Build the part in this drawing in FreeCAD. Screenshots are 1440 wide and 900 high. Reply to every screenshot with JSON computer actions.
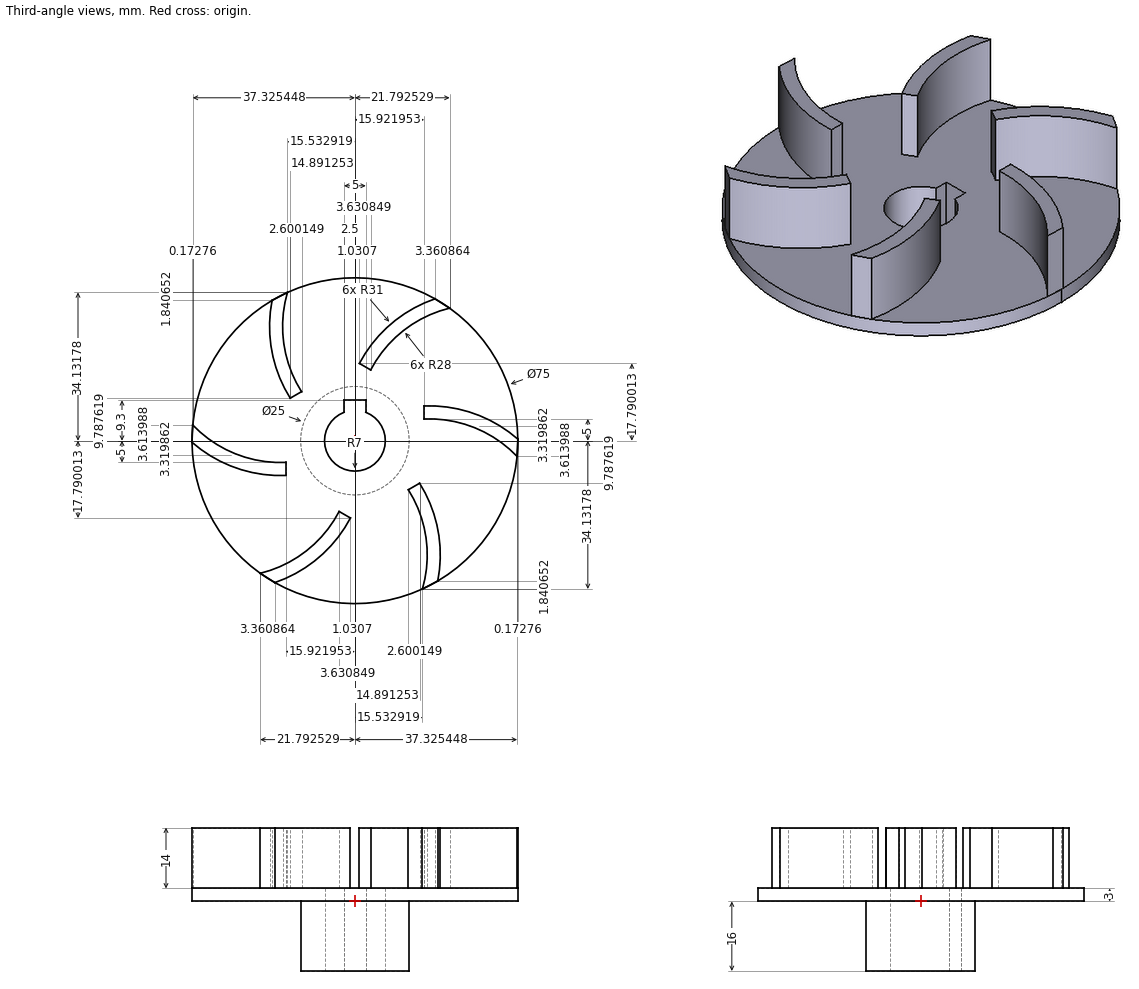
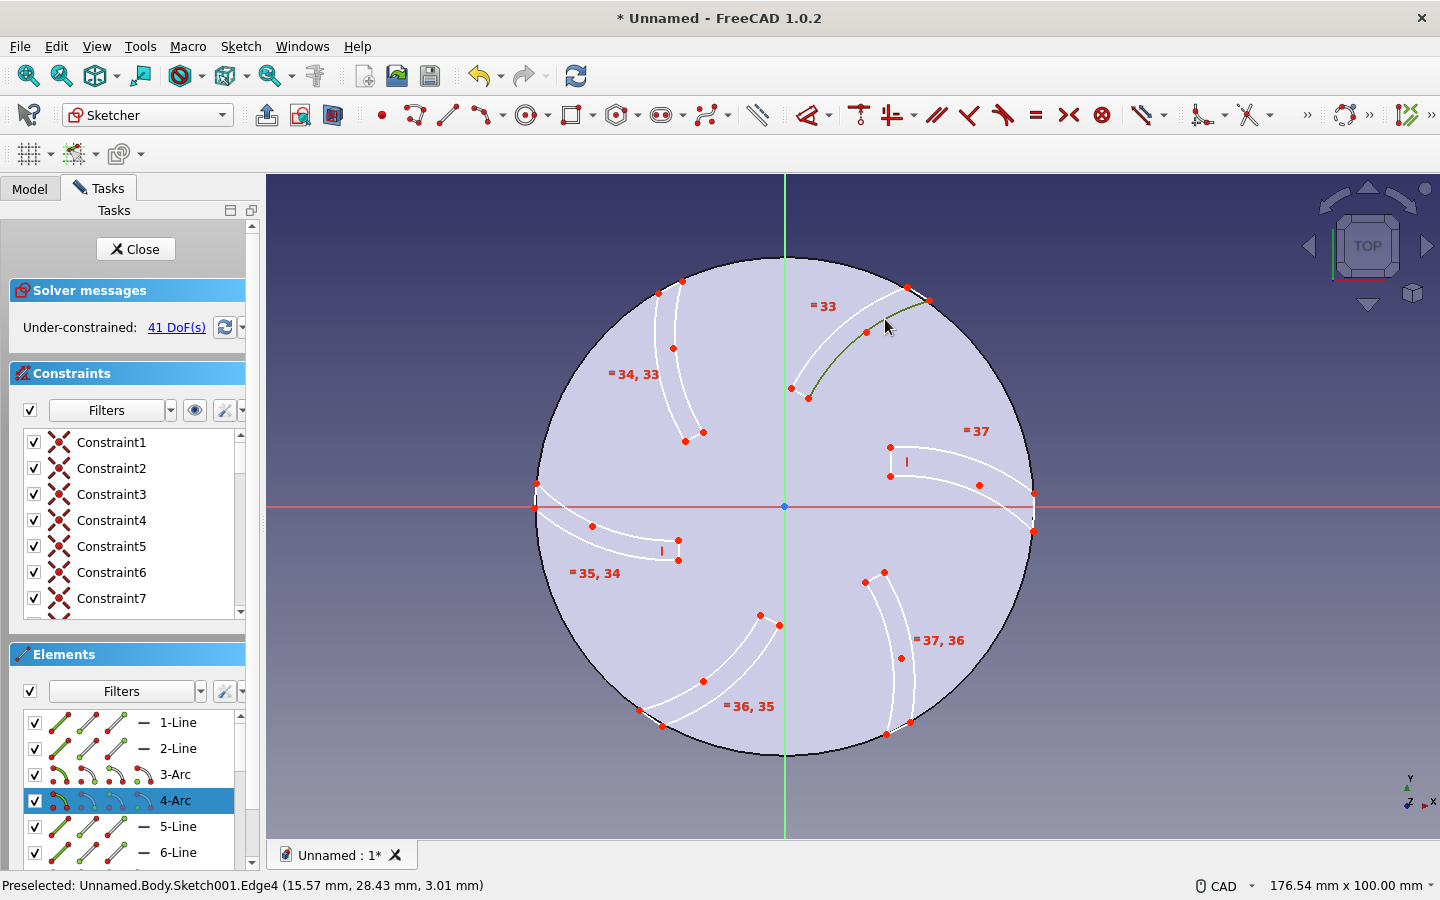
{"action": "left_click", "coordinate": [675, 327]}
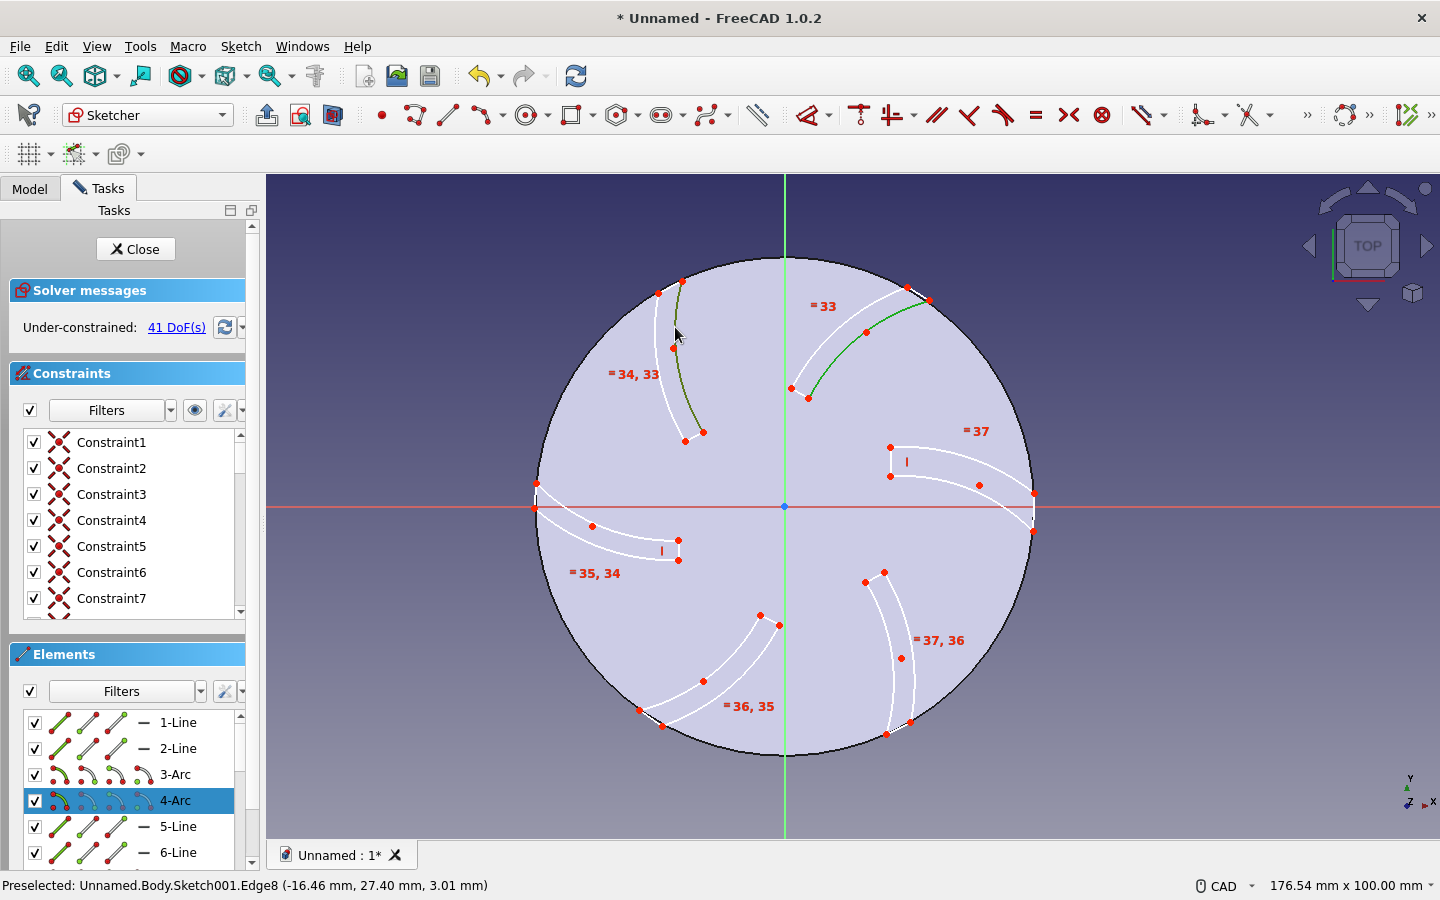
{"action": "left_click", "coordinate": [632, 536]}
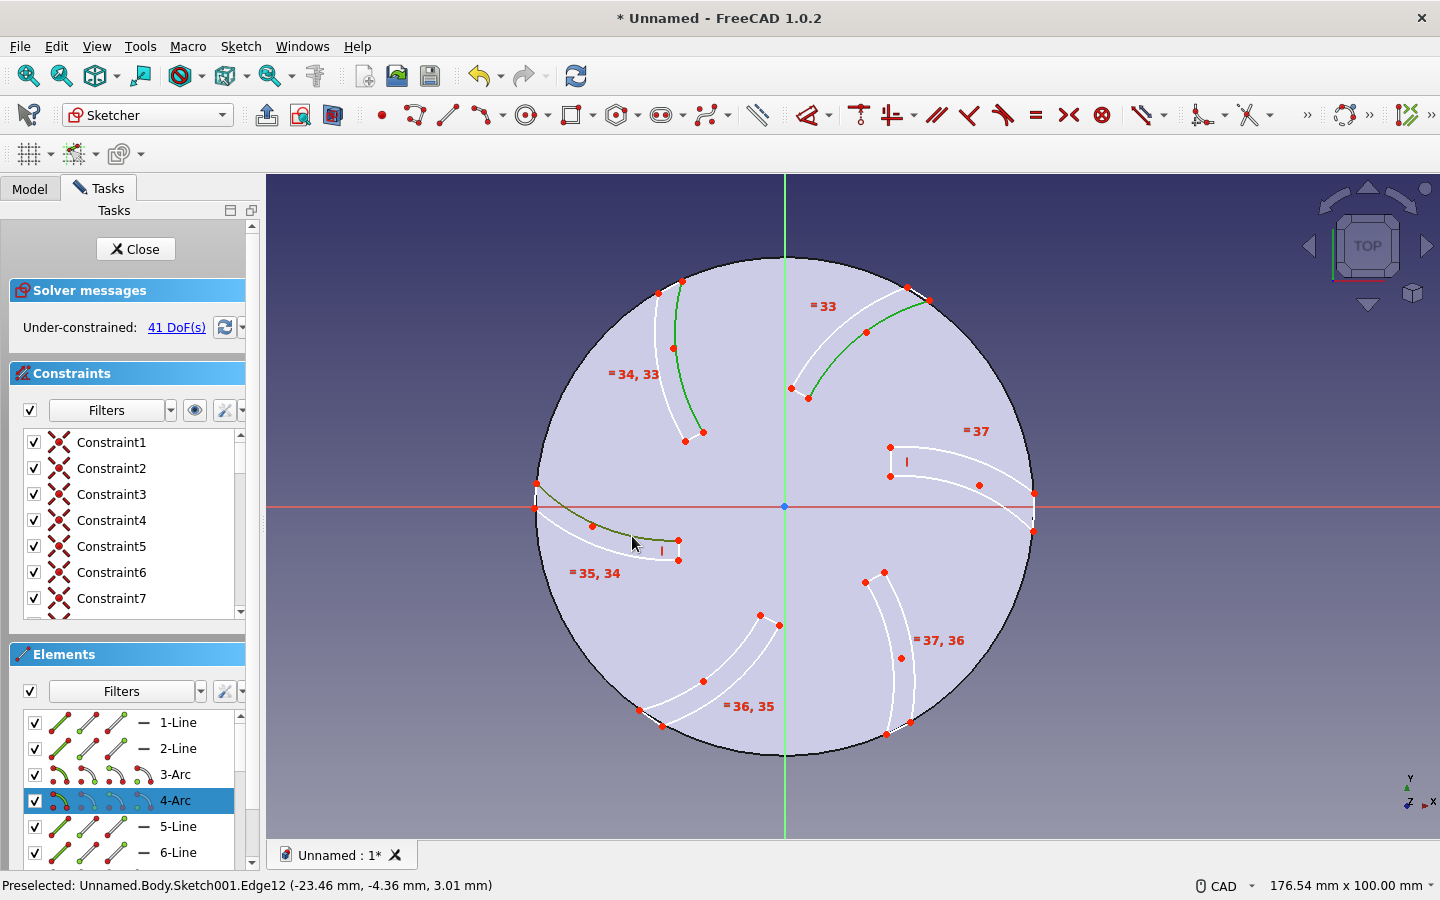
{"action": "left_click", "coordinate": [684, 693]}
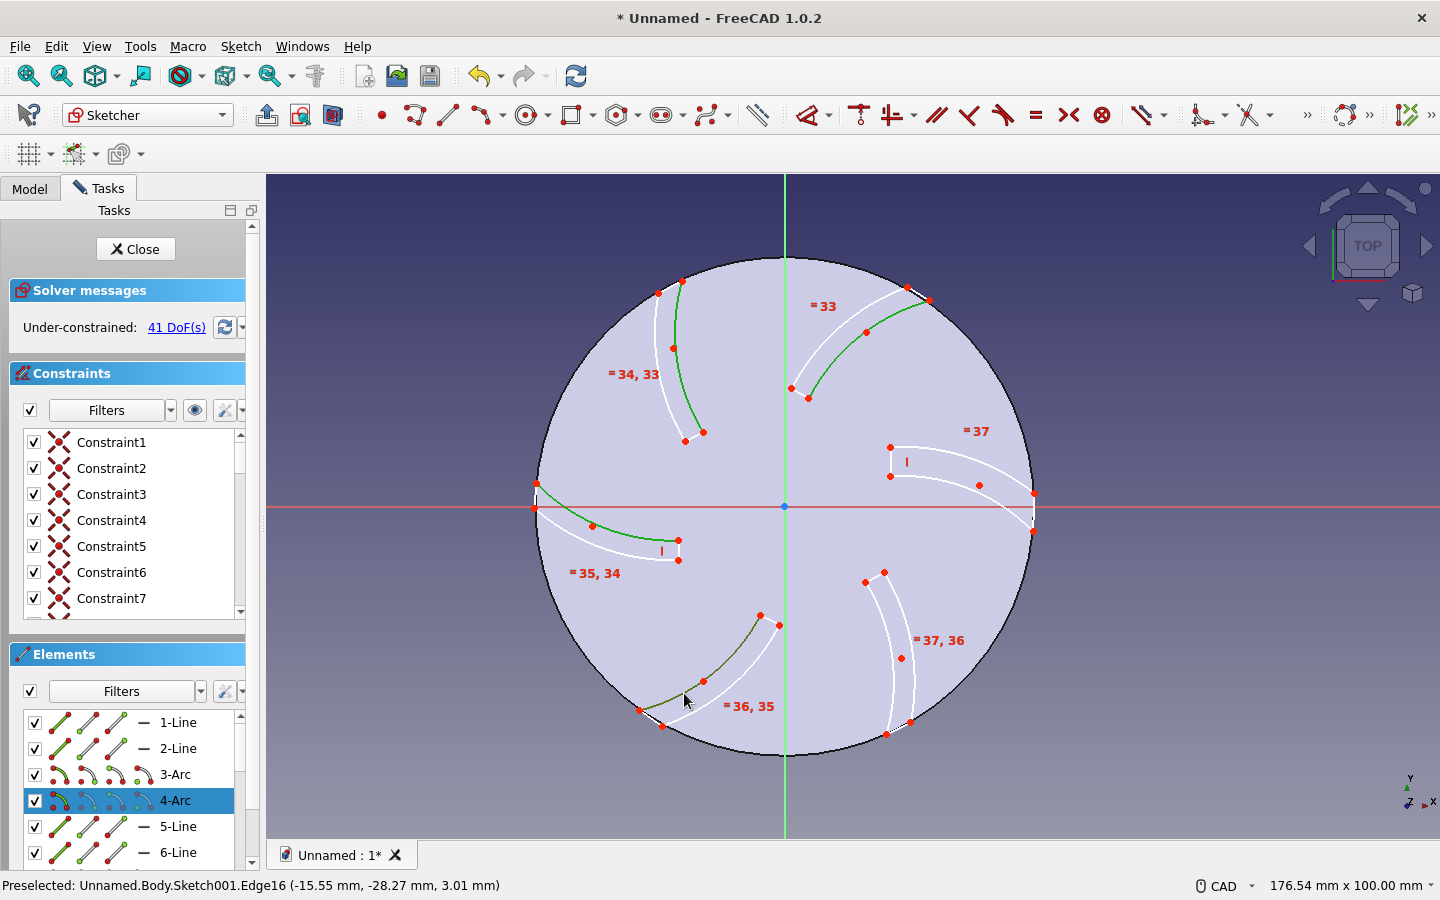
{"action": "left_click", "coordinate": [894, 688]}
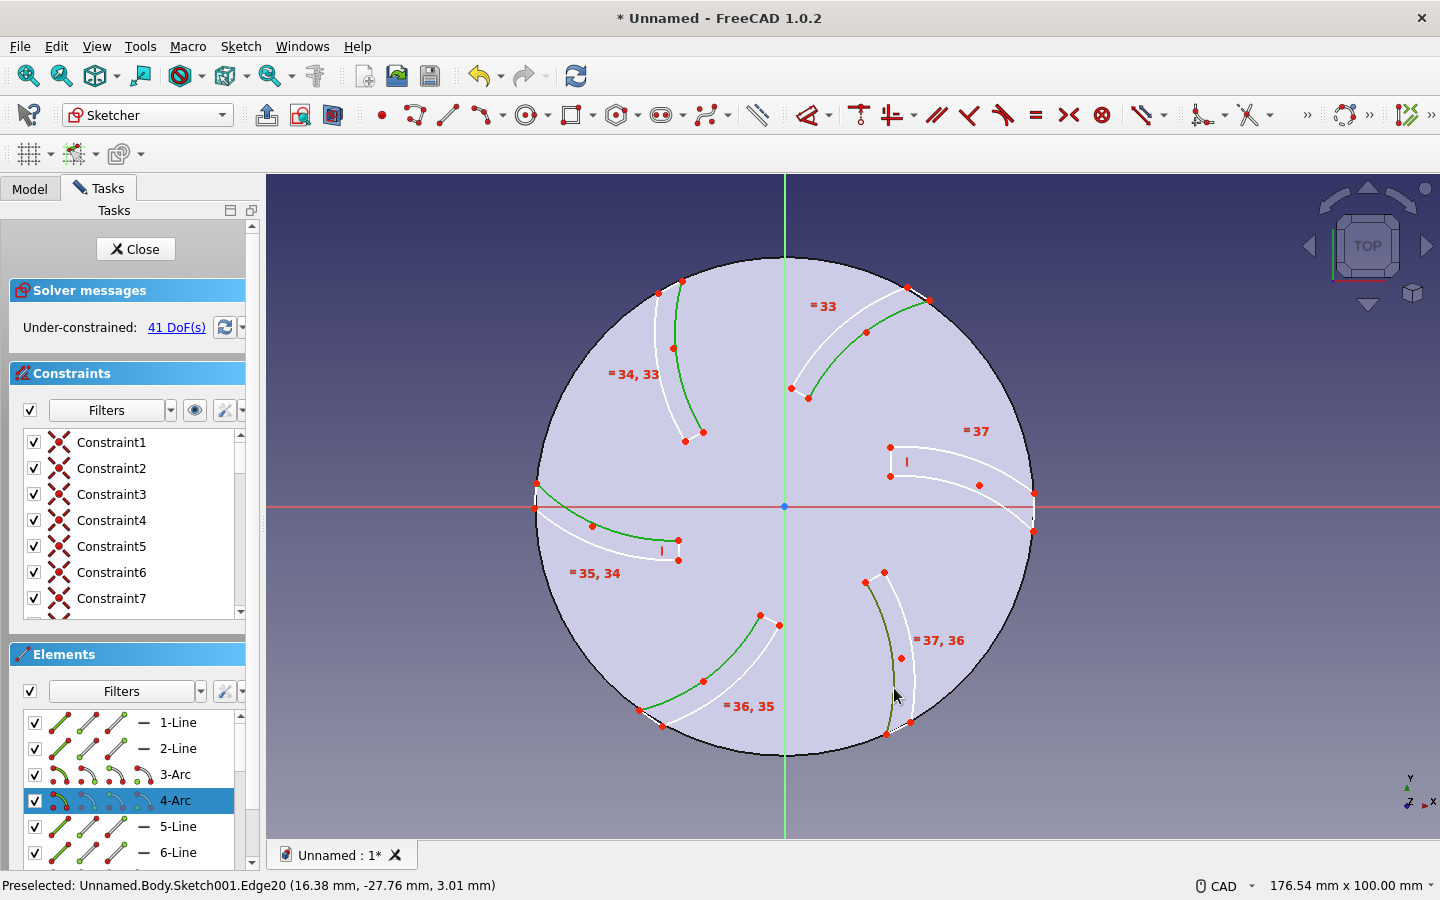
{"action": "left_click", "coordinate": [938, 480]}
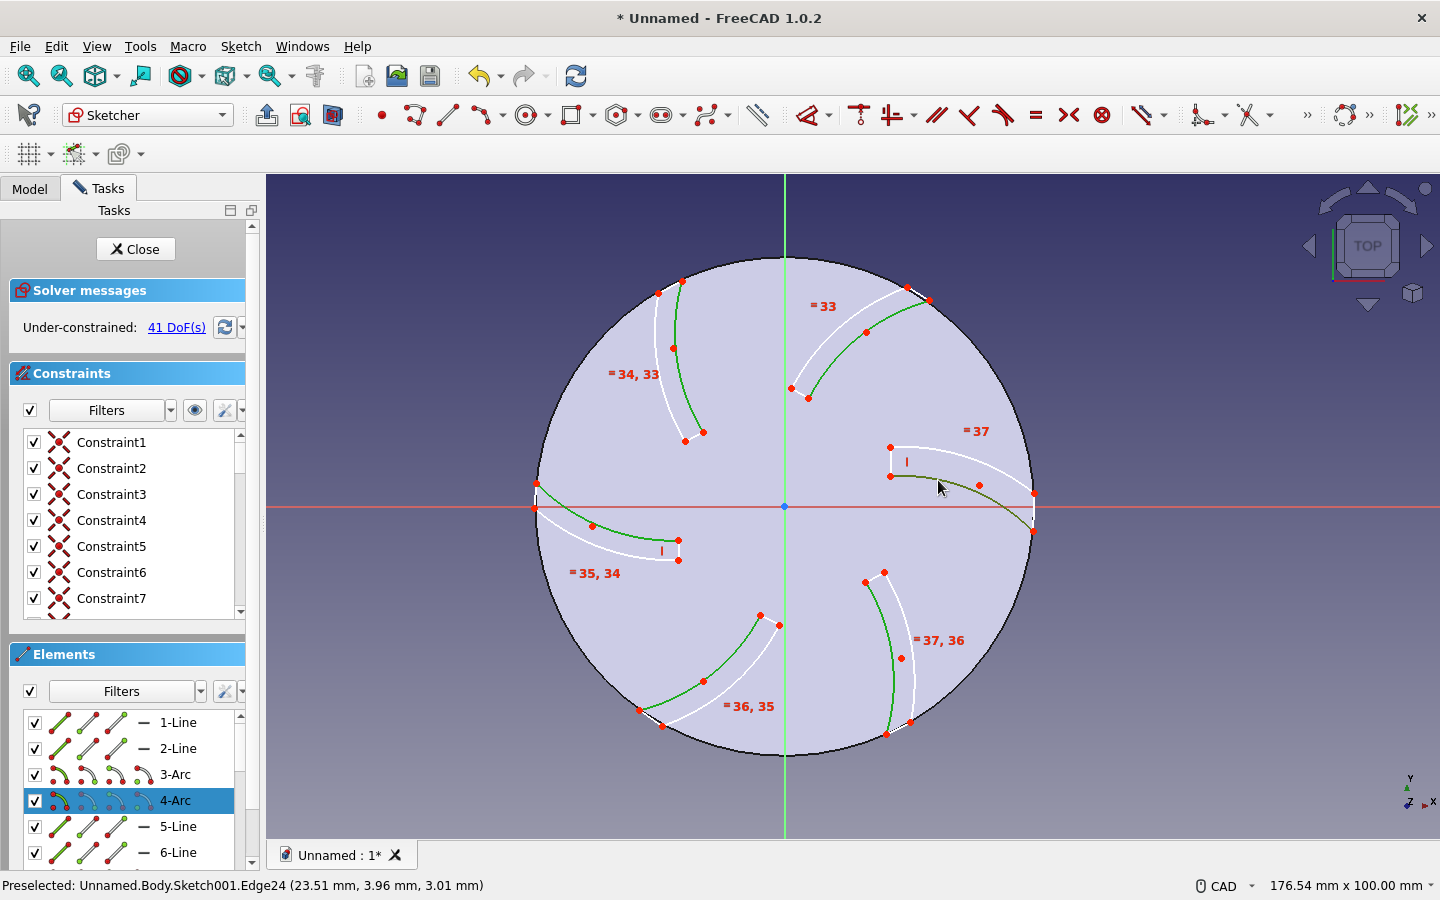
{"action": "key", "text": "e"}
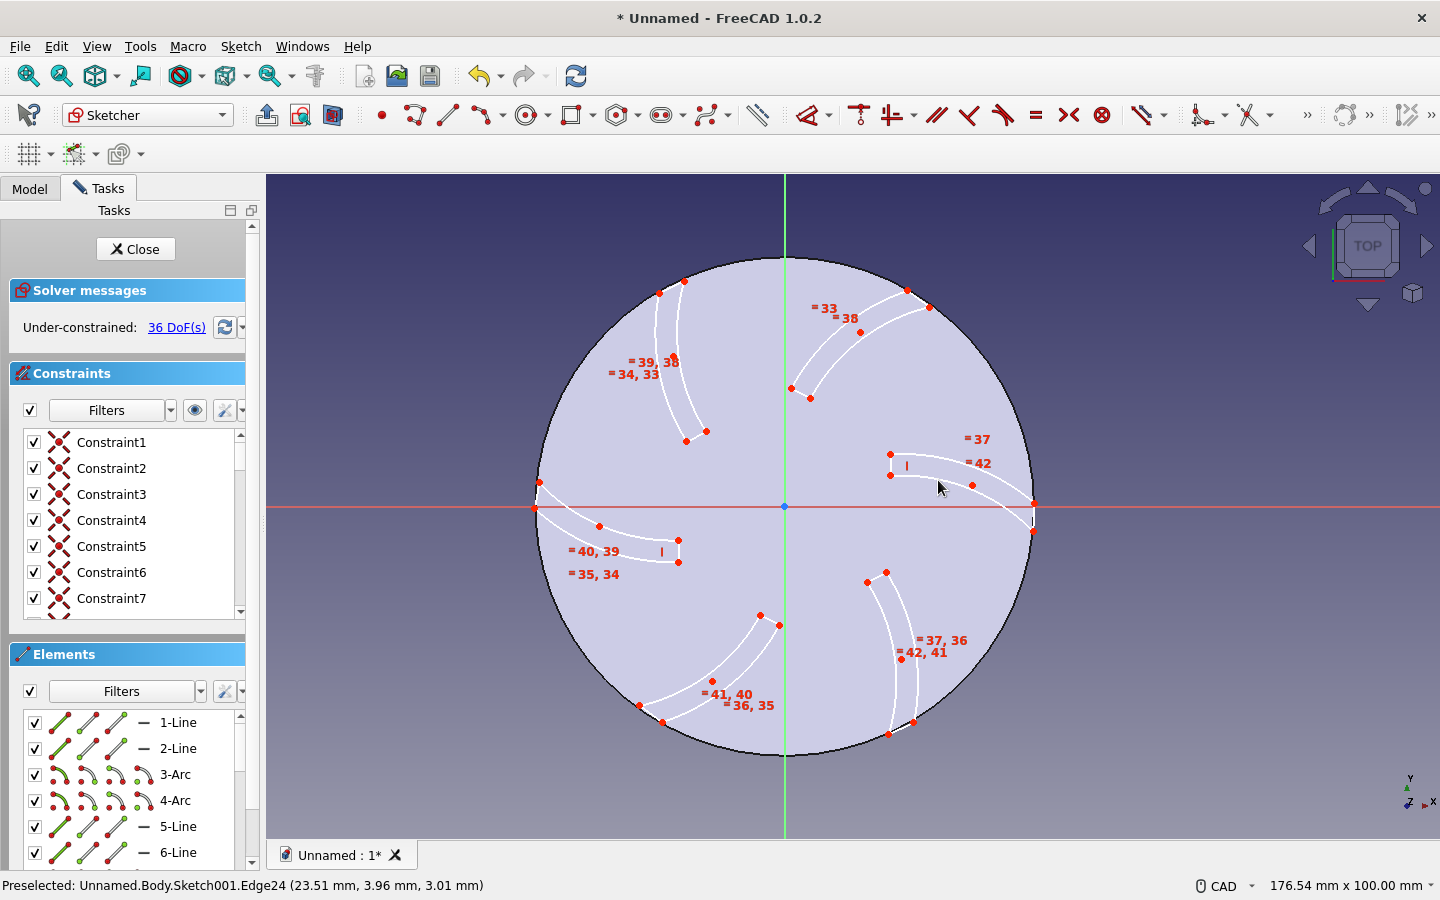
{"action": "left_click", "coordinate": [865, 310]}